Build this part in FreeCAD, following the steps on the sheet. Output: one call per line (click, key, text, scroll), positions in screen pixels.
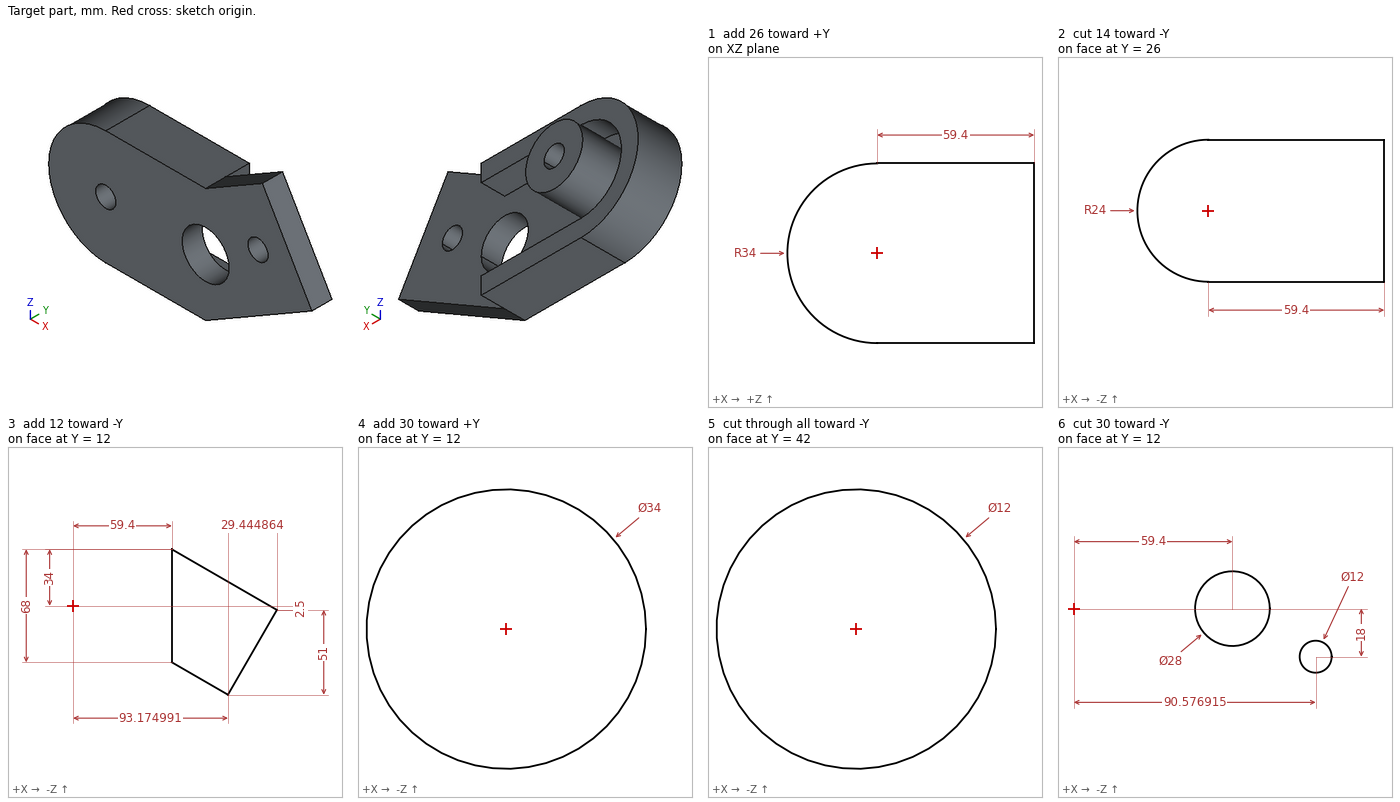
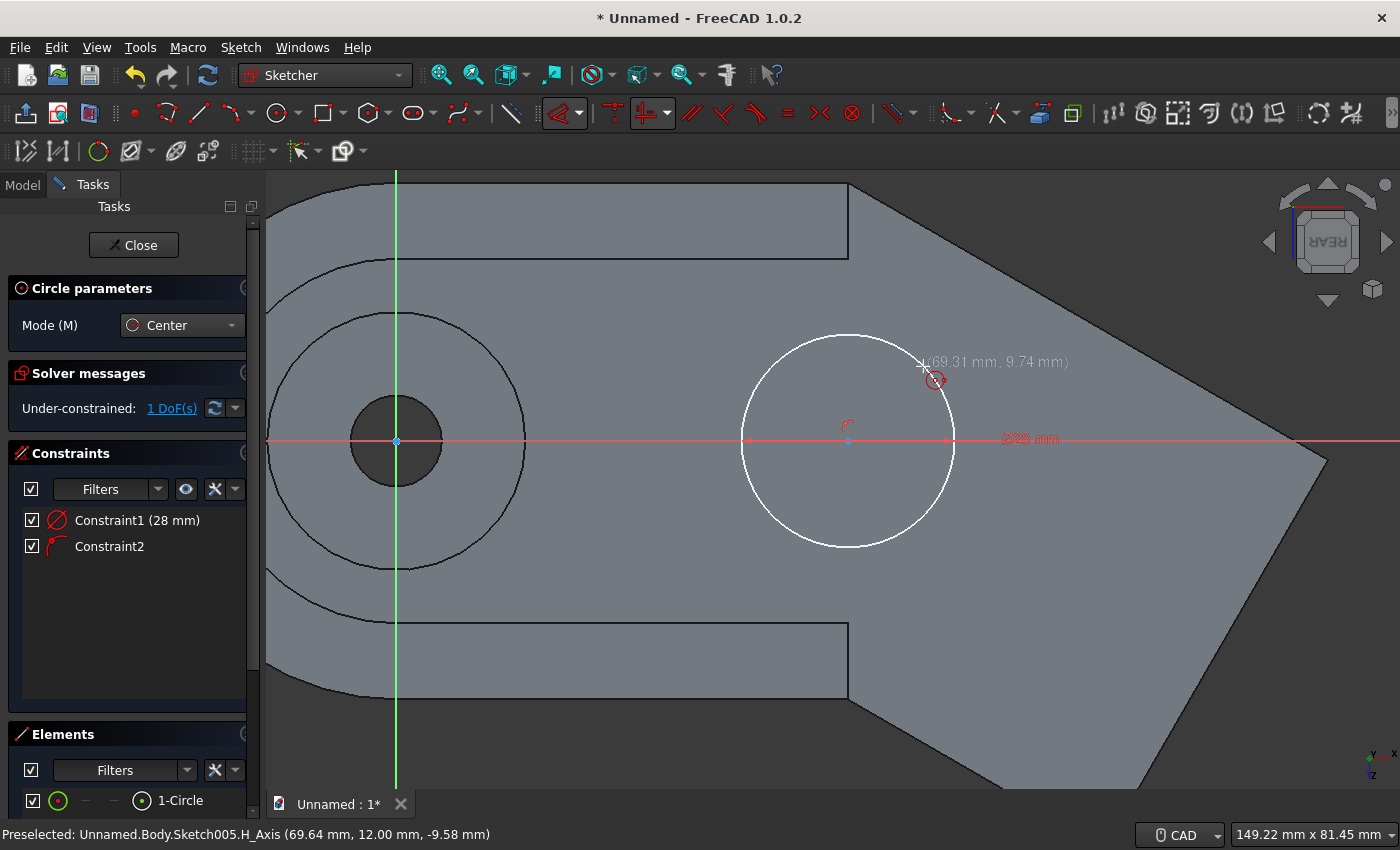
click(1085, 578)
move(1117, 546)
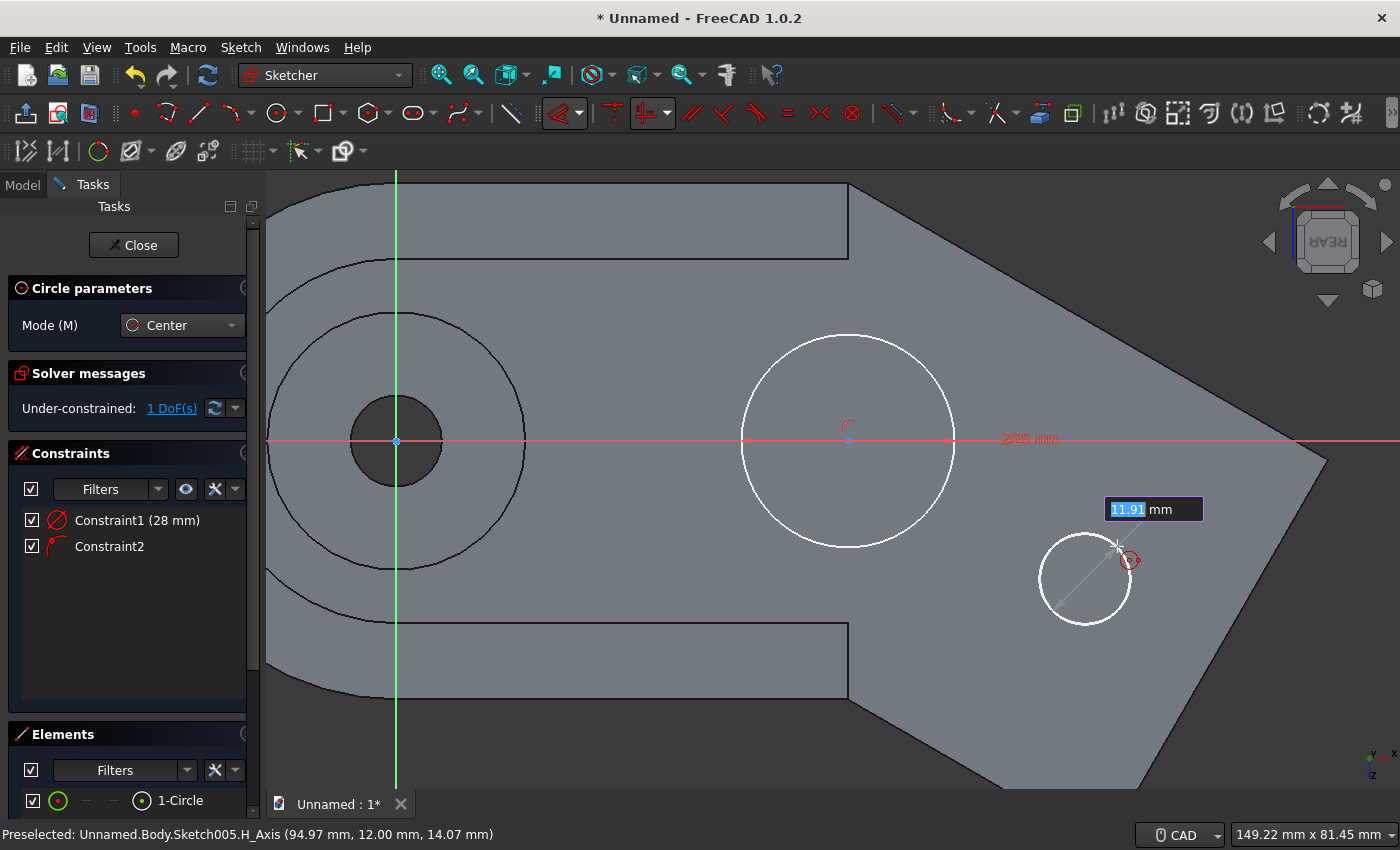
text(12)
key(Return)
key(Escape)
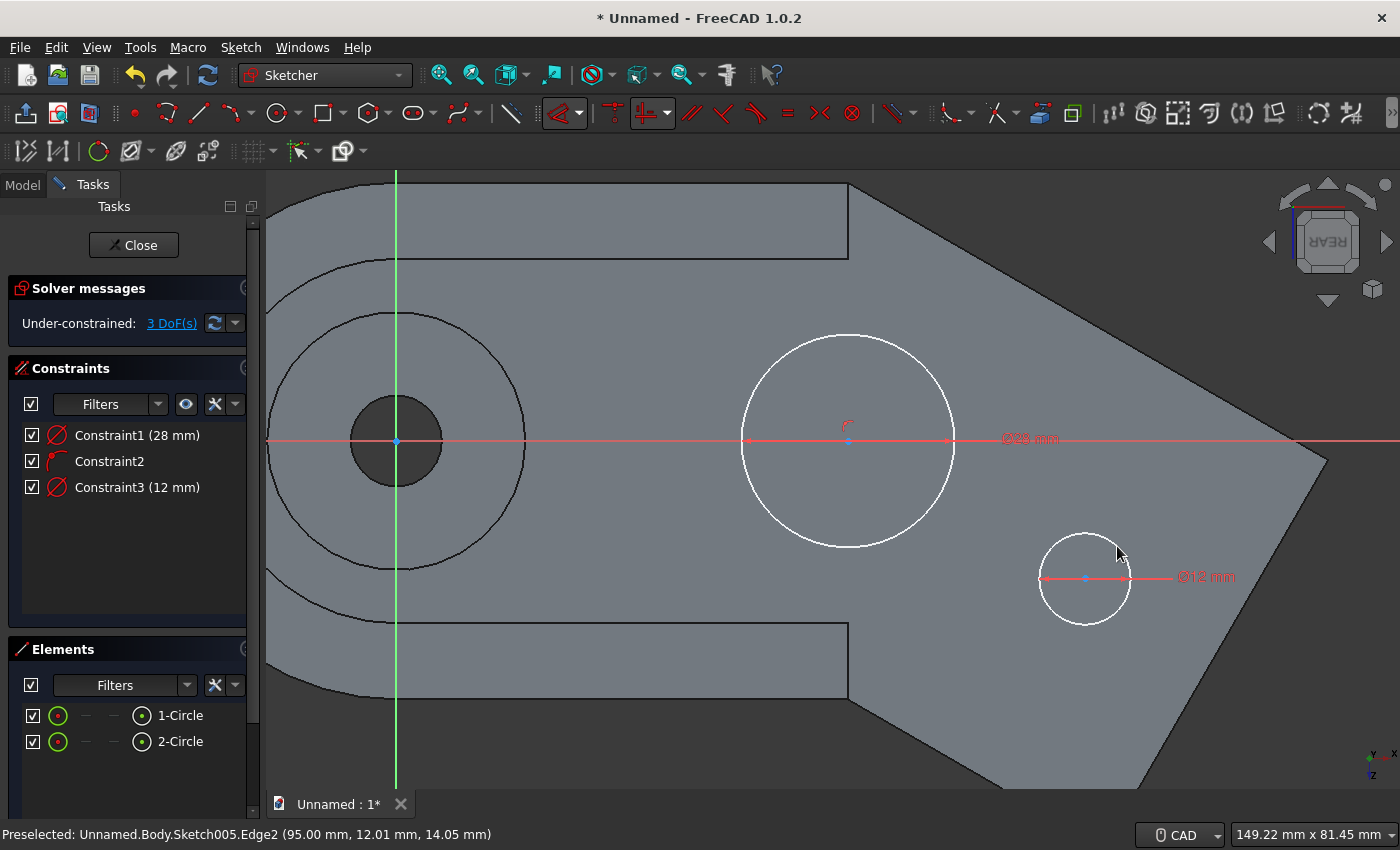
click(1085, 579)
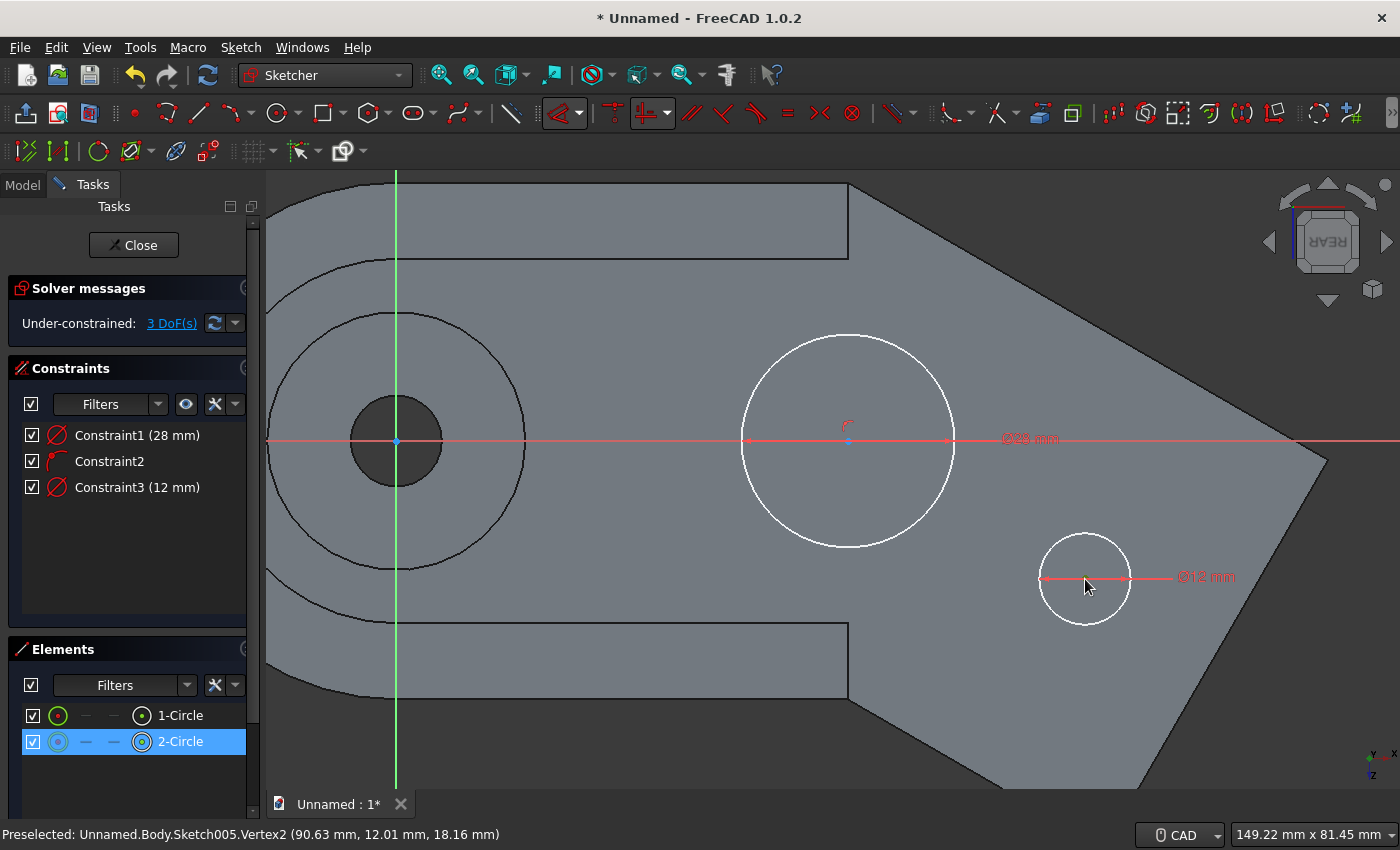
click(582, 114)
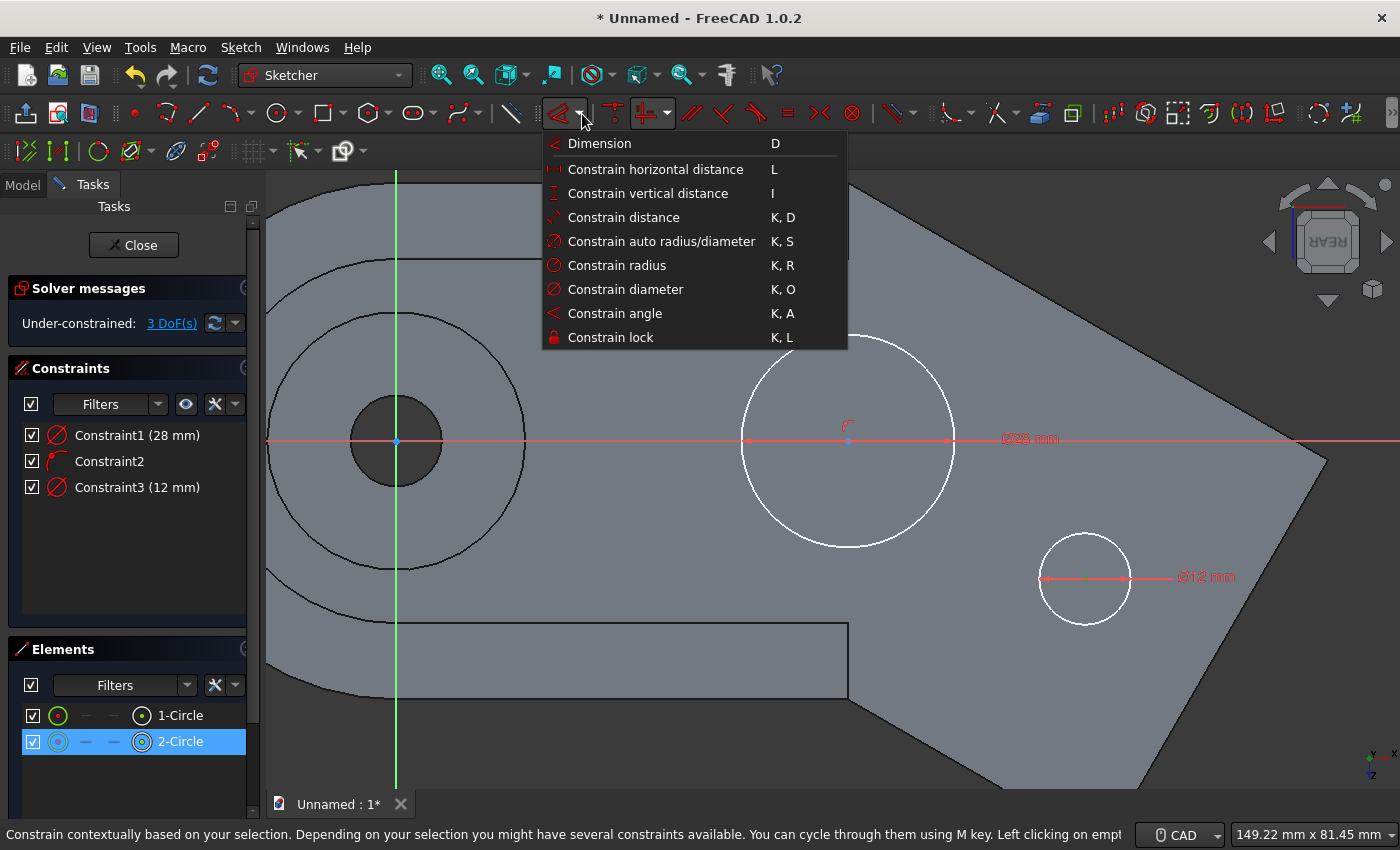
click(695, 193)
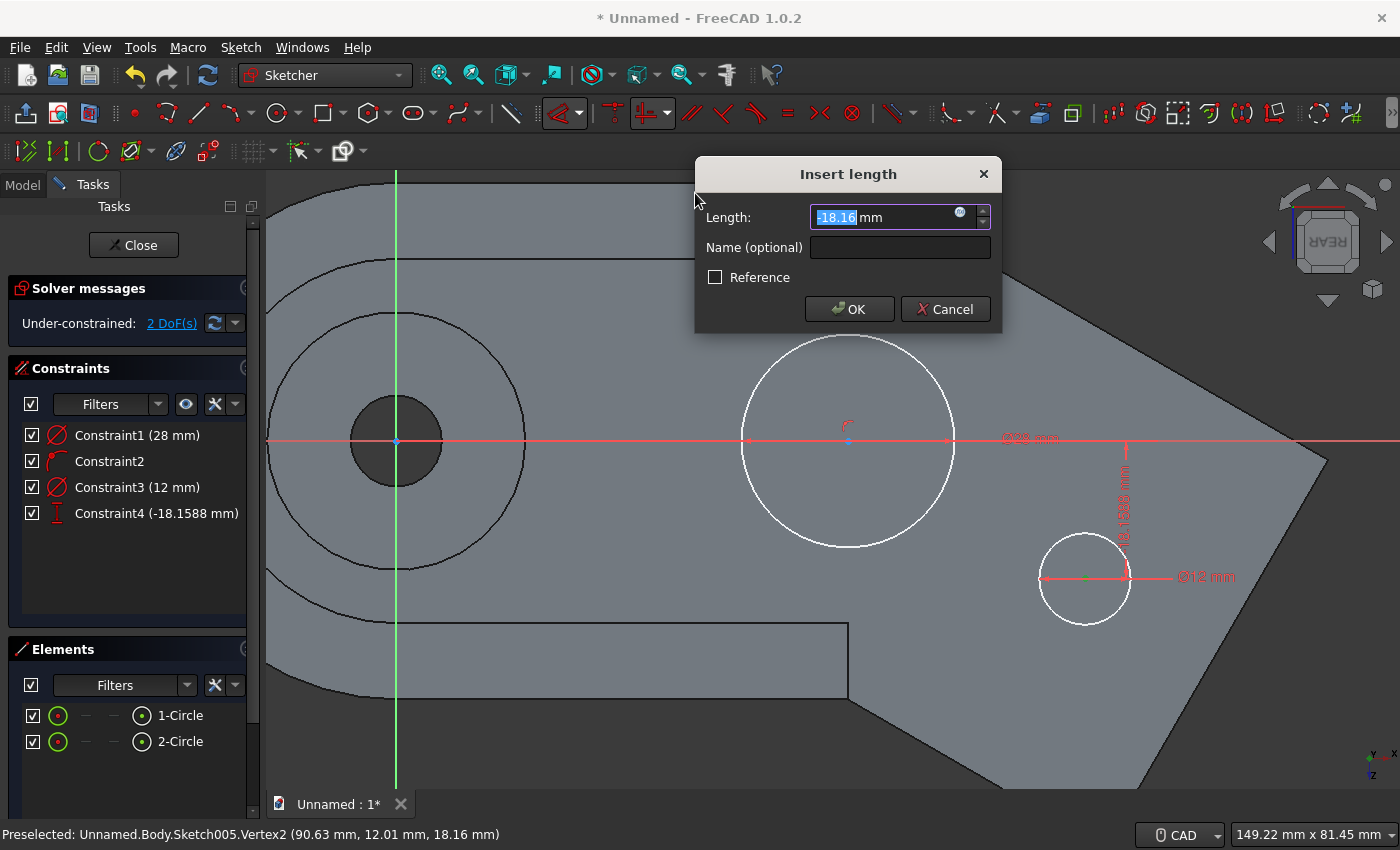
text(-18)
key(Return)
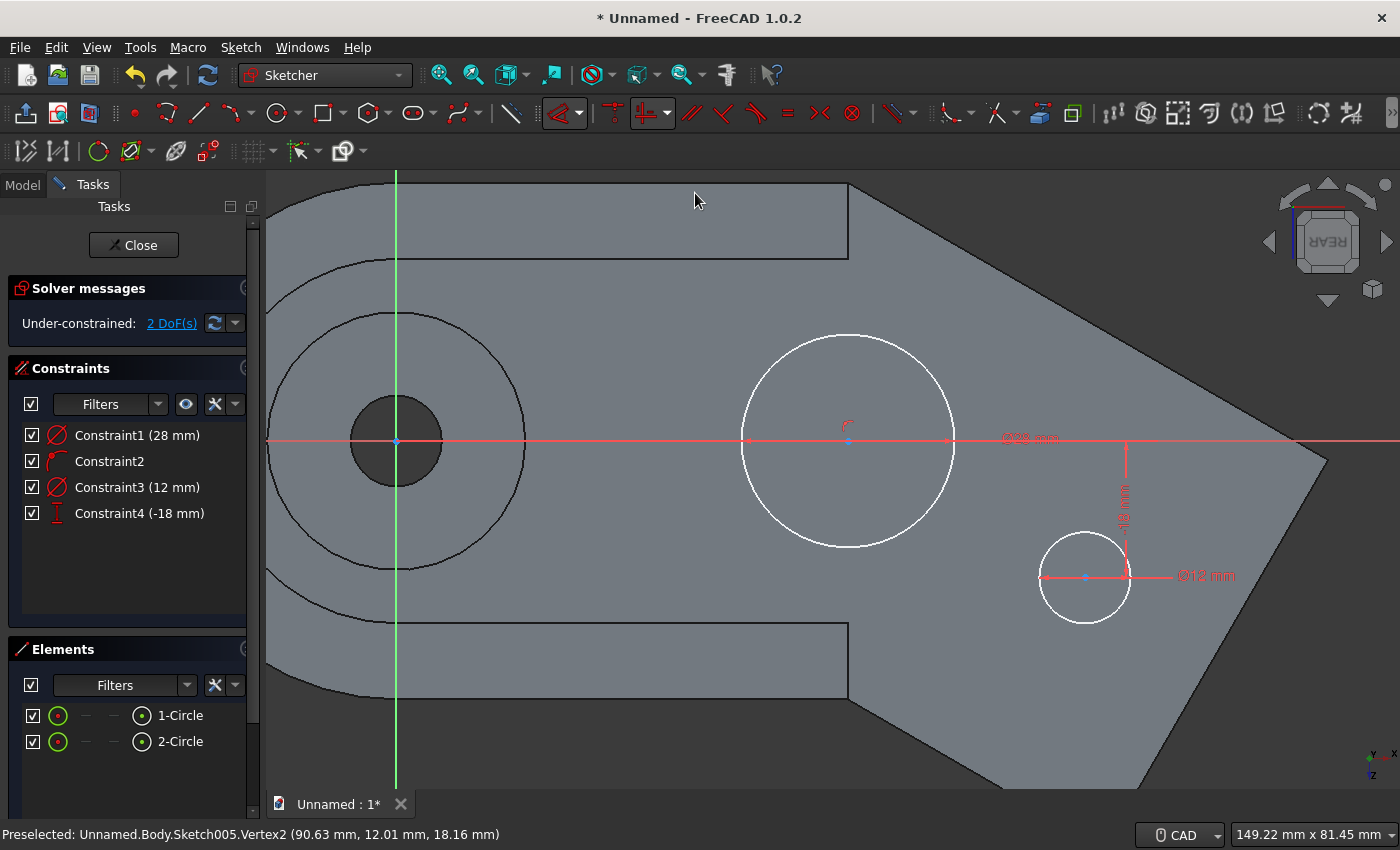
click(848, 441)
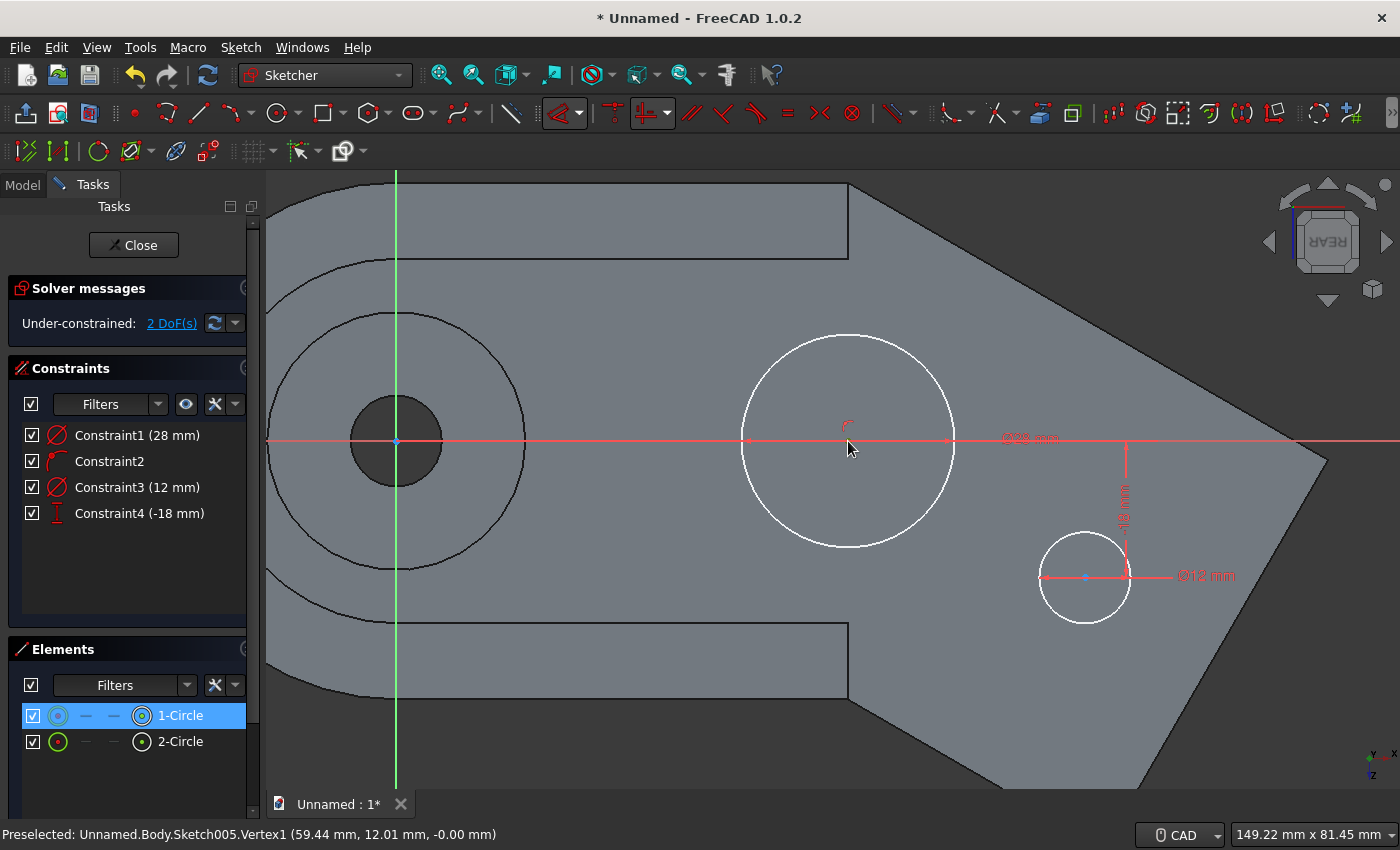
key(l)